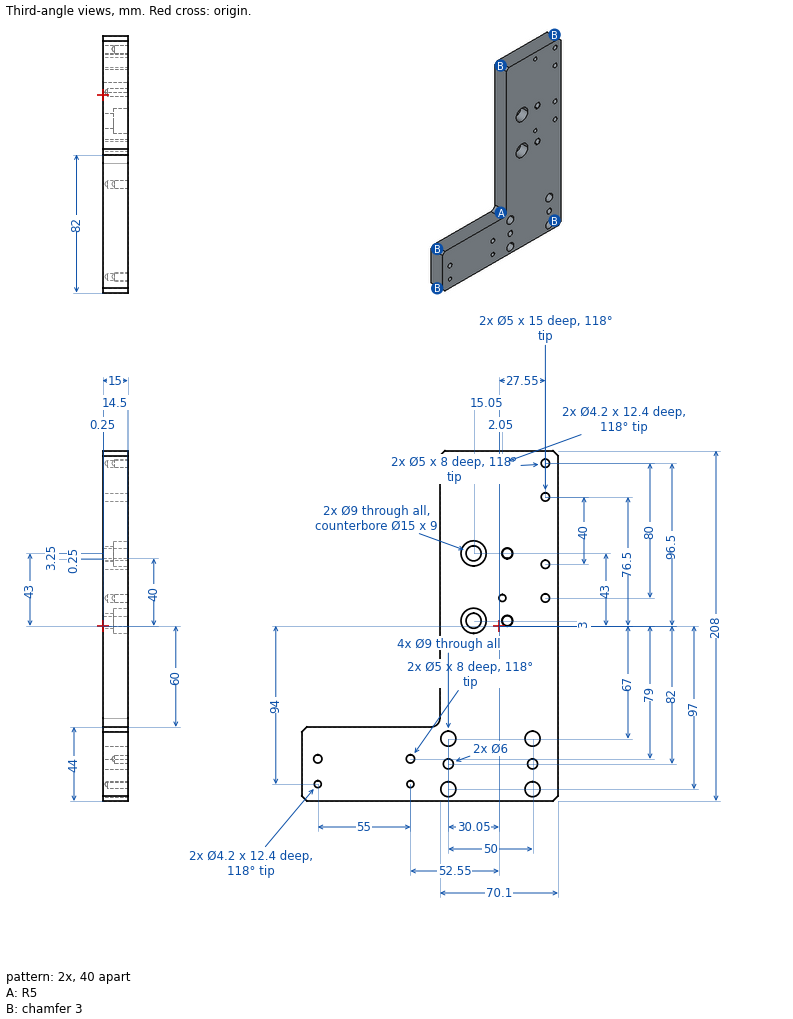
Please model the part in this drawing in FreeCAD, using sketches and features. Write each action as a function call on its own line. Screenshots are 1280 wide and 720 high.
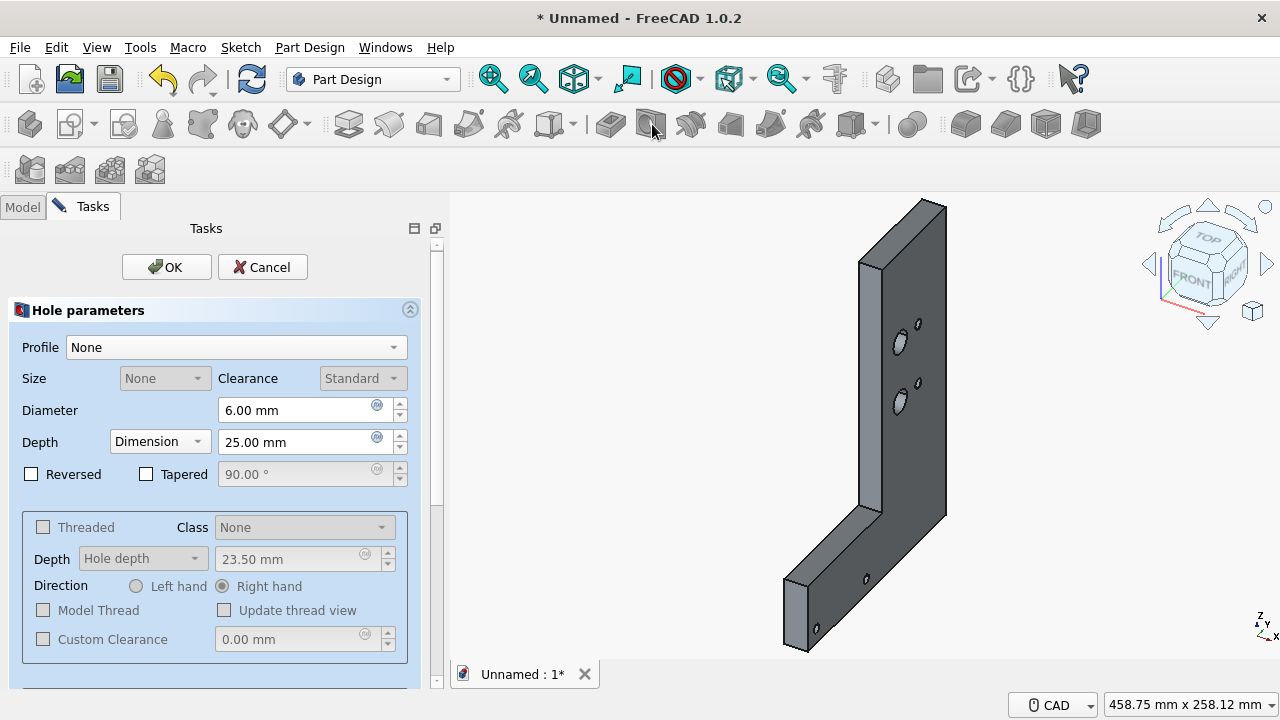
triple_click(305, 410)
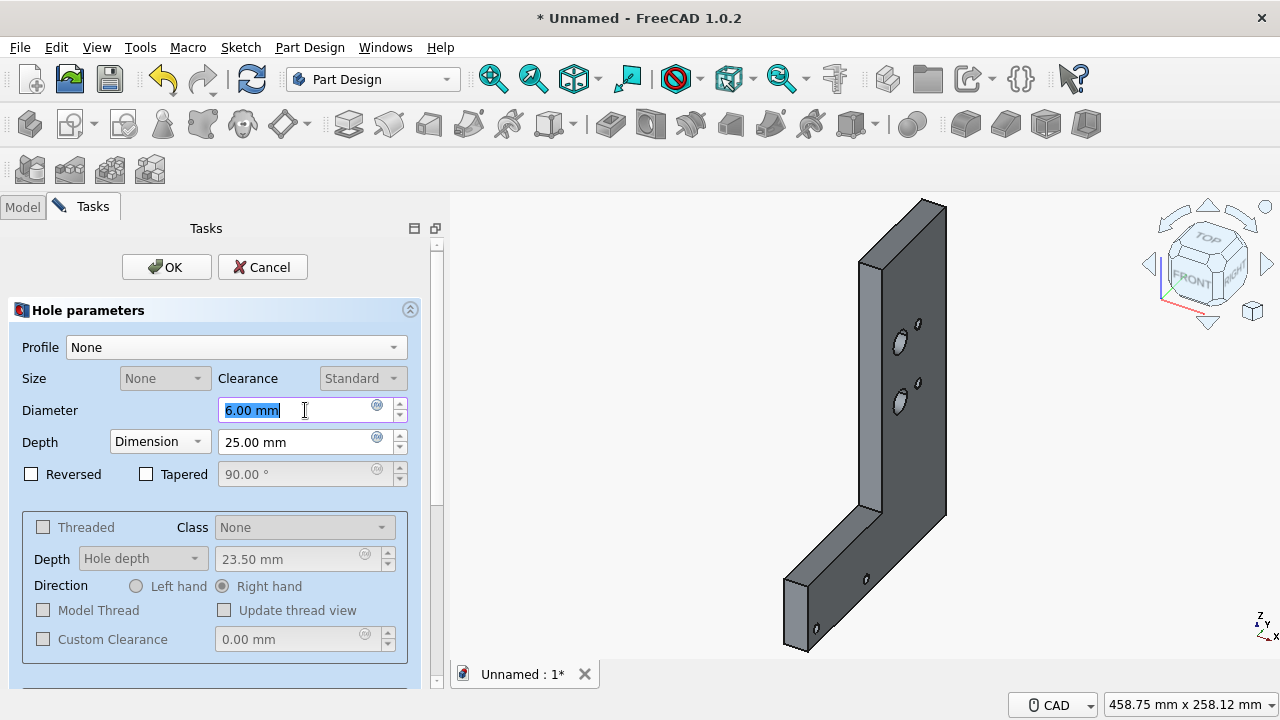
text(4.2)
key(Tab)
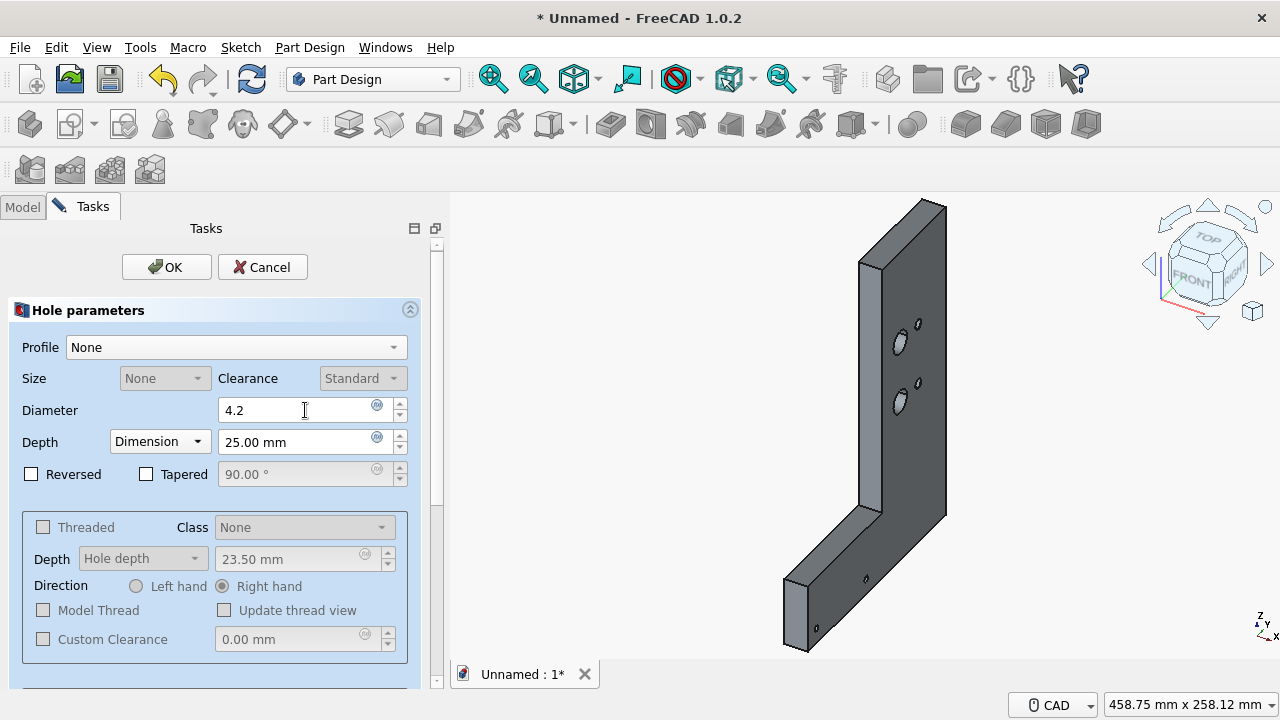
triple_click(305, 442)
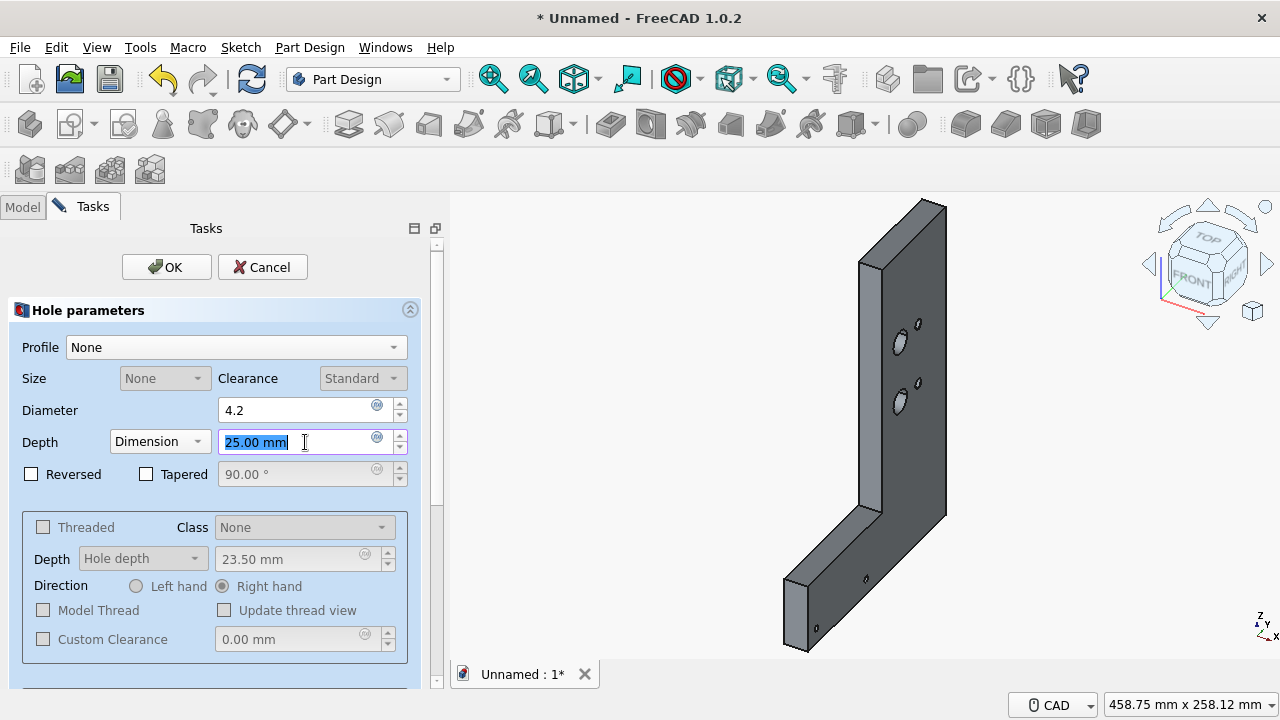
text(12.4)
key(Tab)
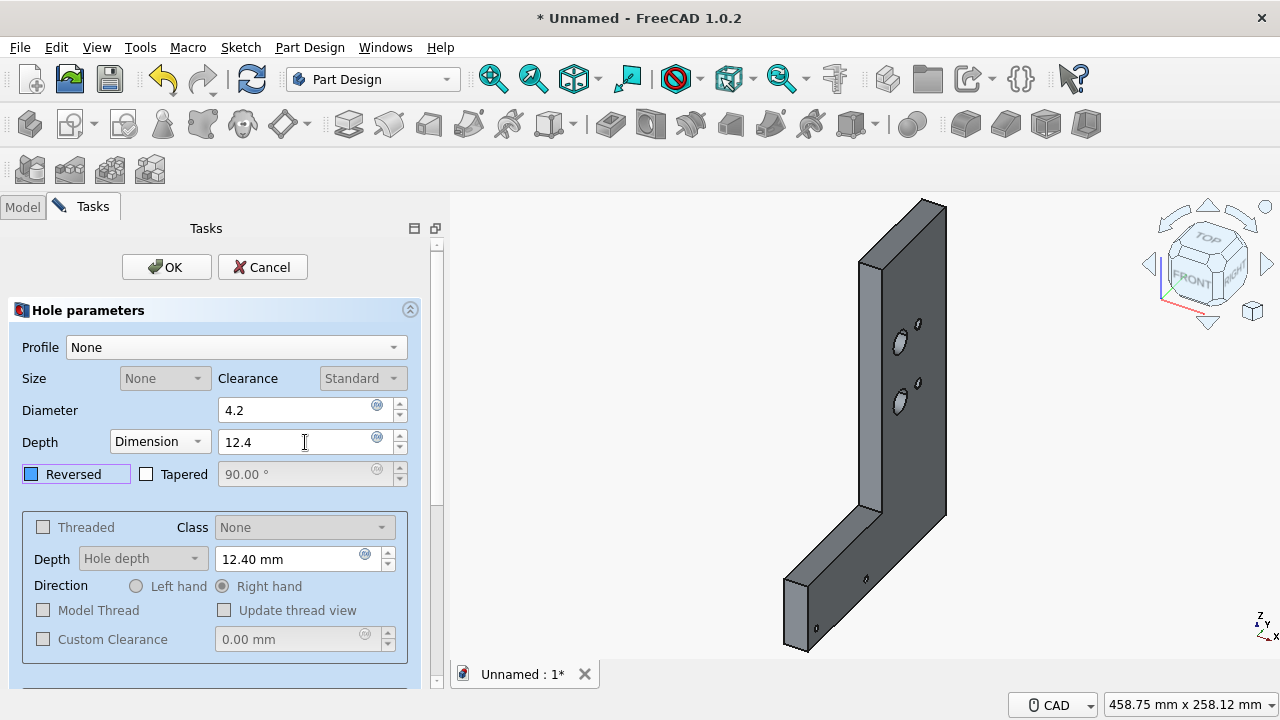
click(167, 267)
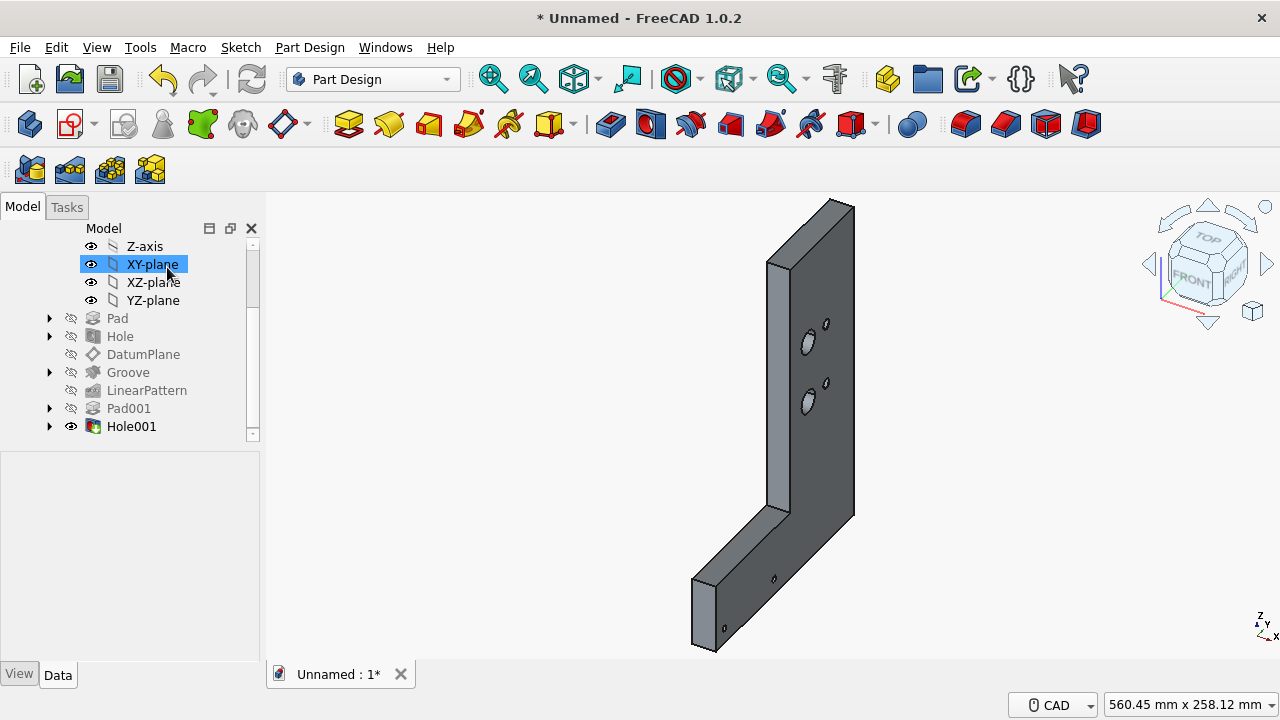
click(824, 477)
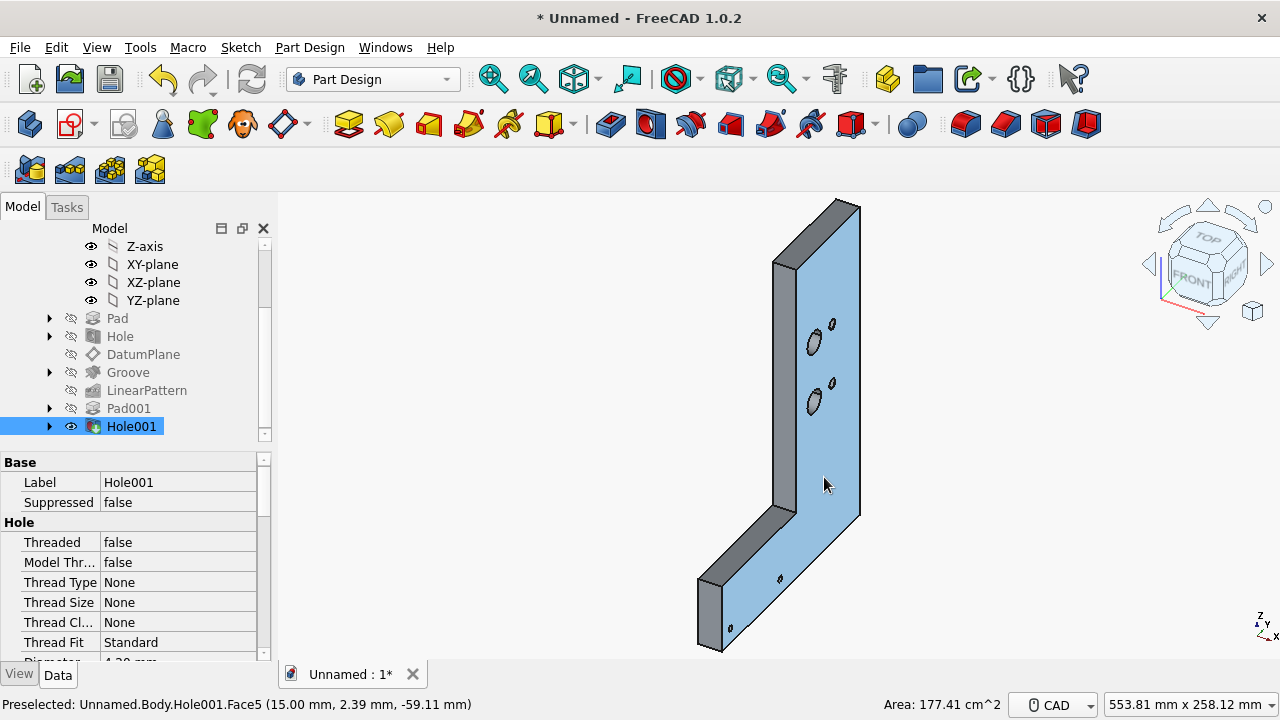
click(70, 124)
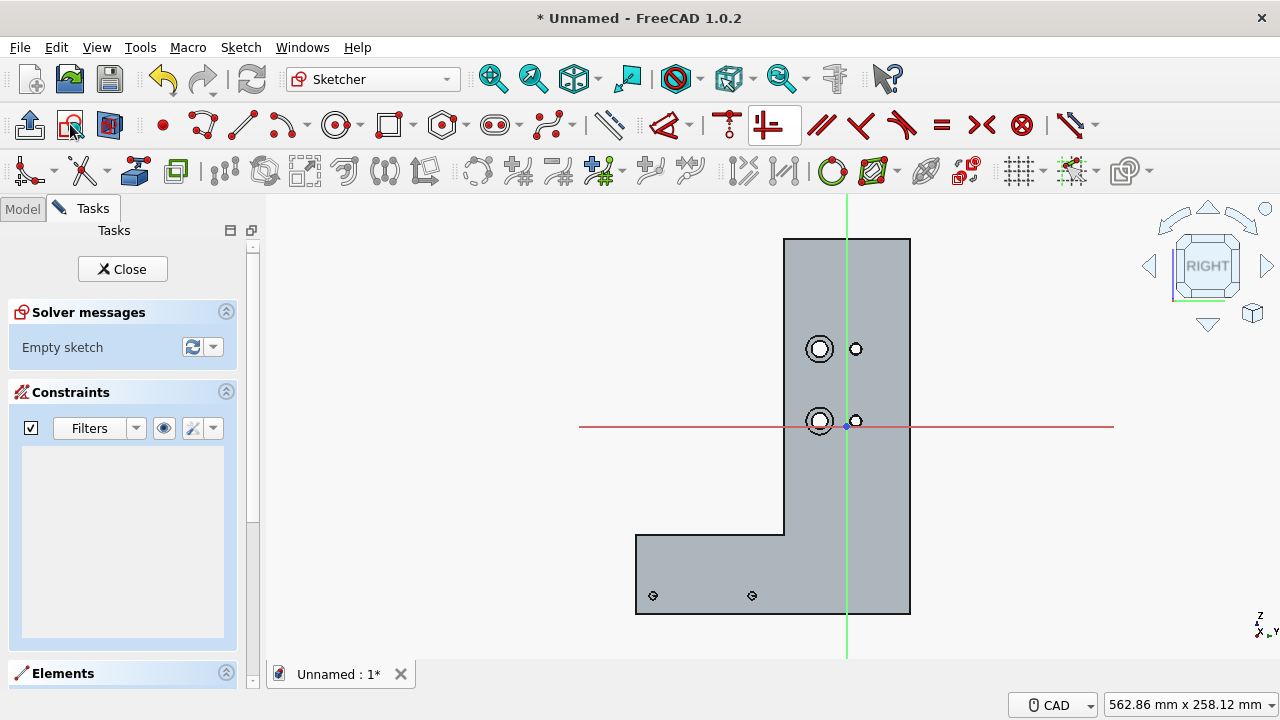
scroll(800, 589, up, 3)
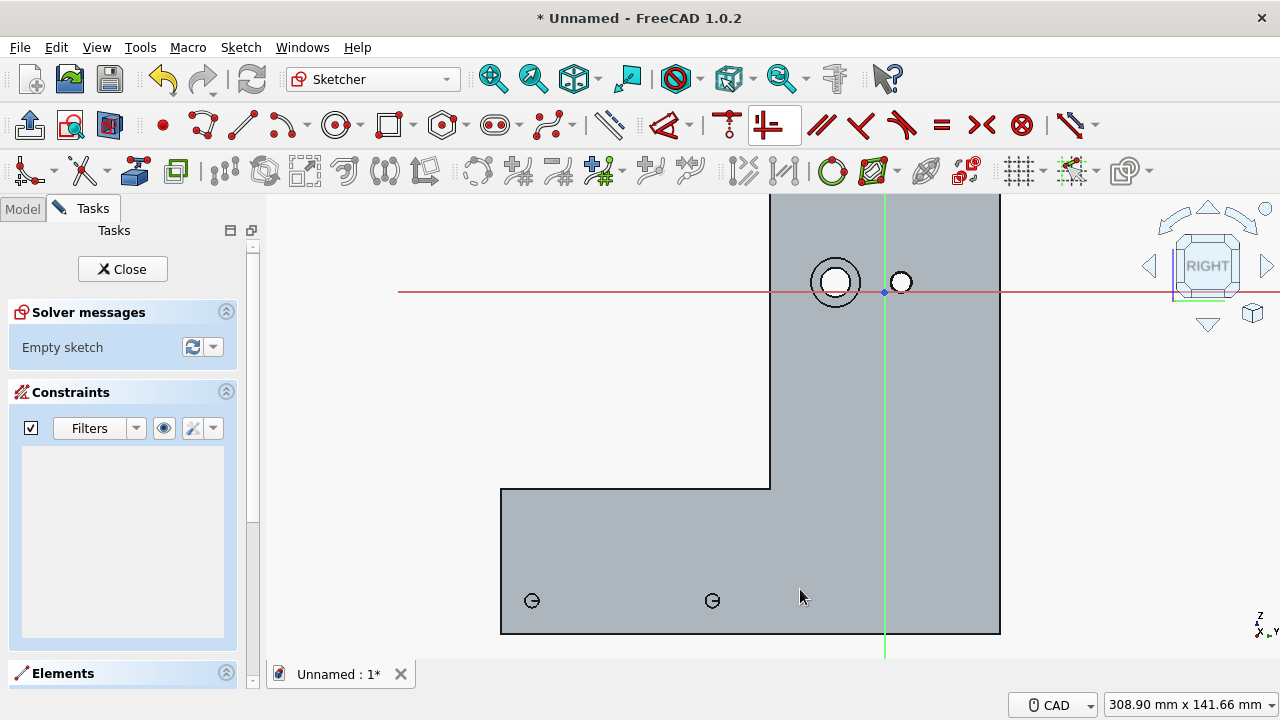
key(g)
key(c)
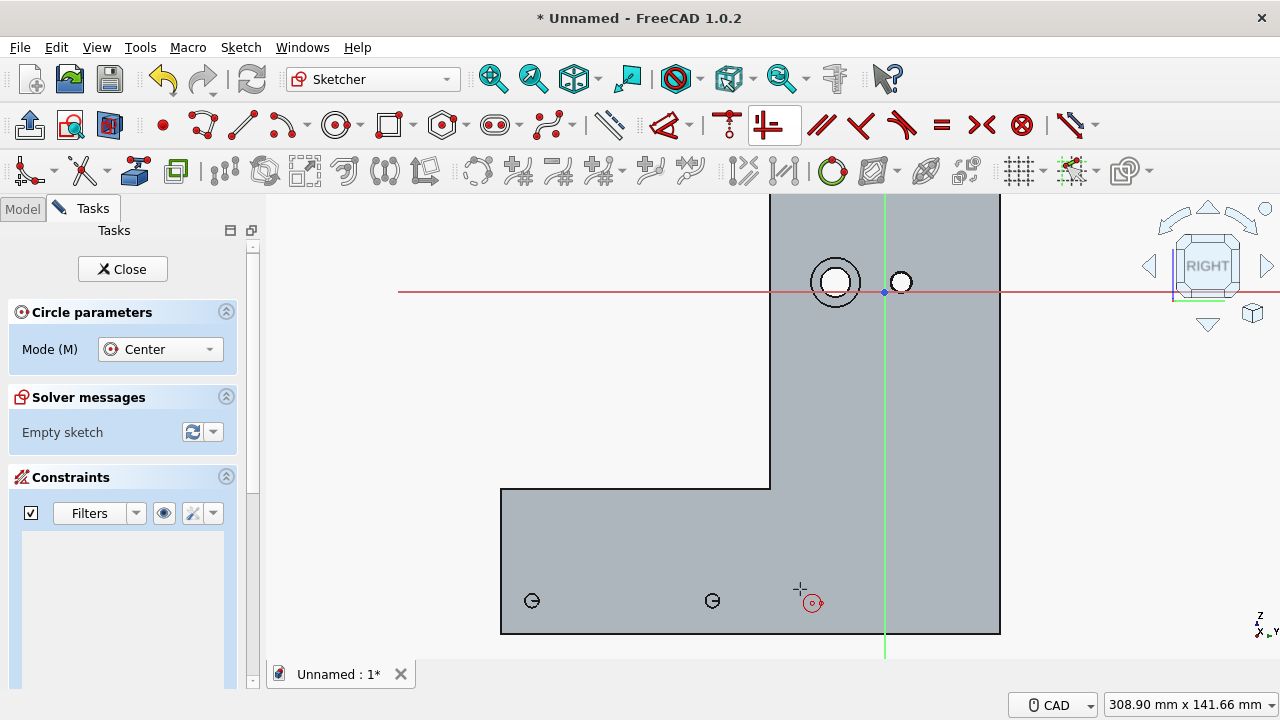
scroll(712, 552, up, 6)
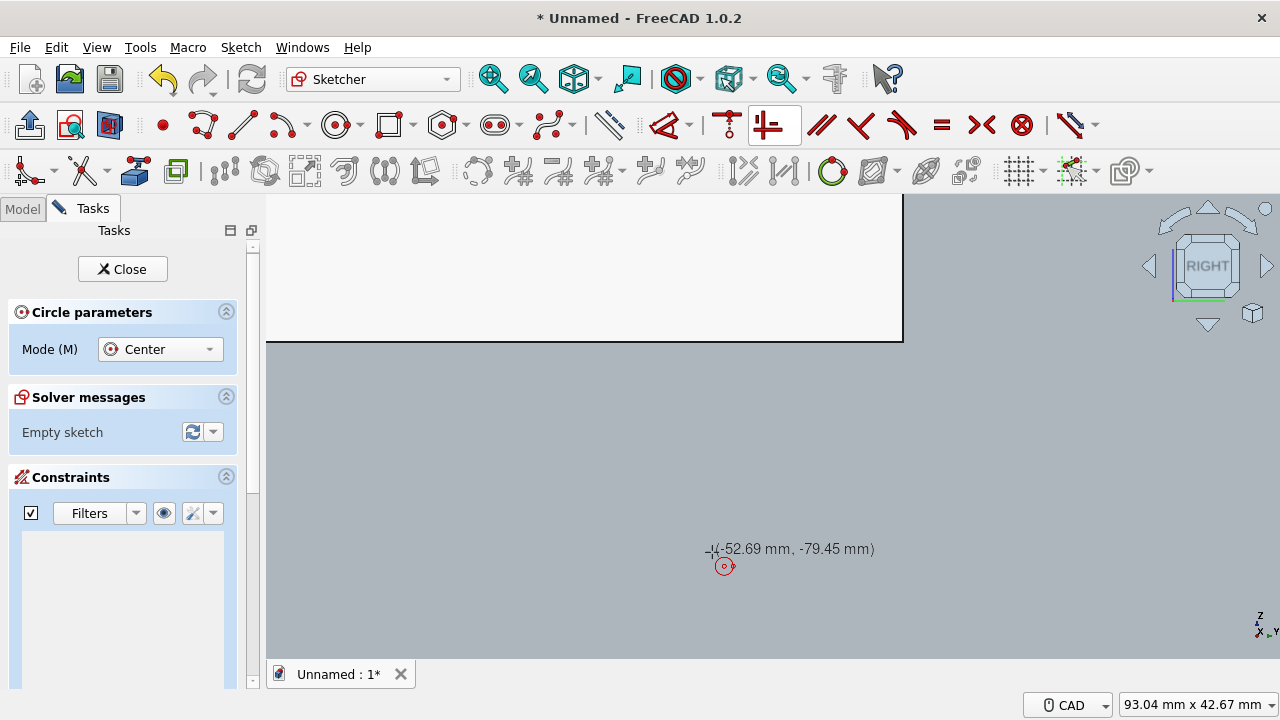
click(712, 549)
click(732, 529)